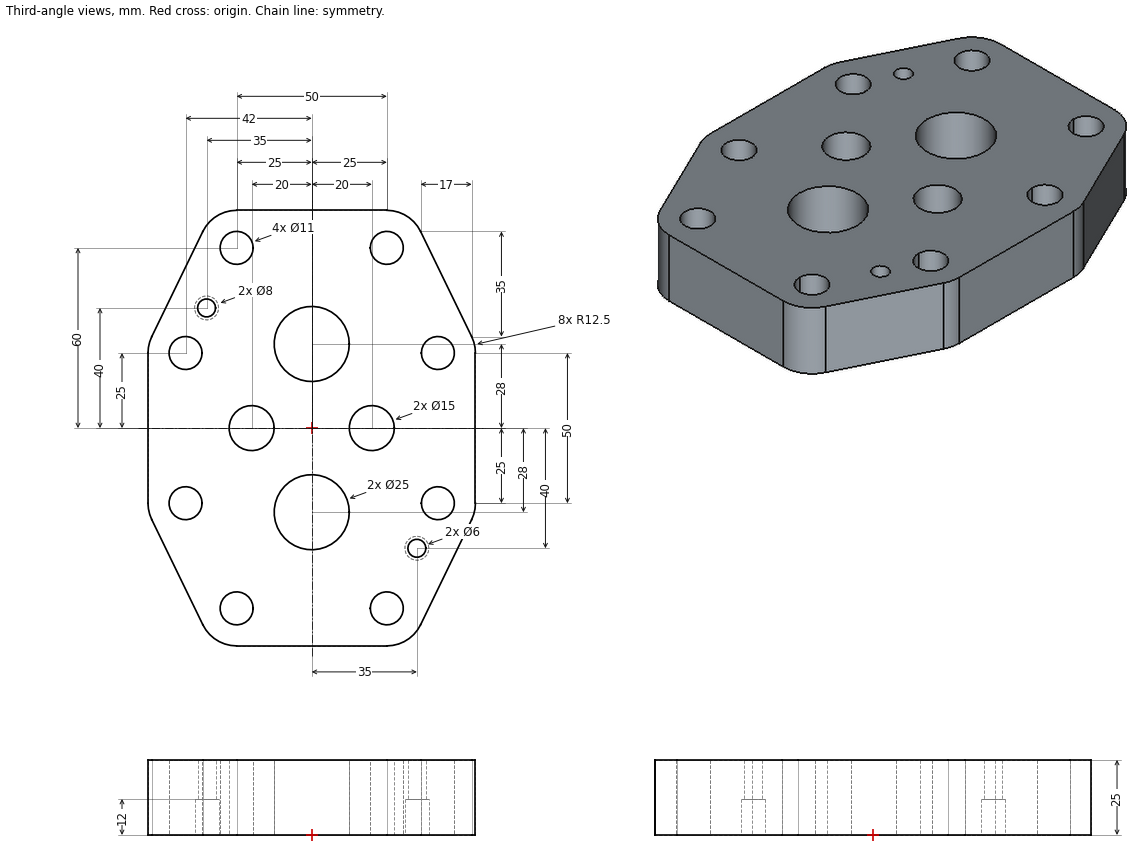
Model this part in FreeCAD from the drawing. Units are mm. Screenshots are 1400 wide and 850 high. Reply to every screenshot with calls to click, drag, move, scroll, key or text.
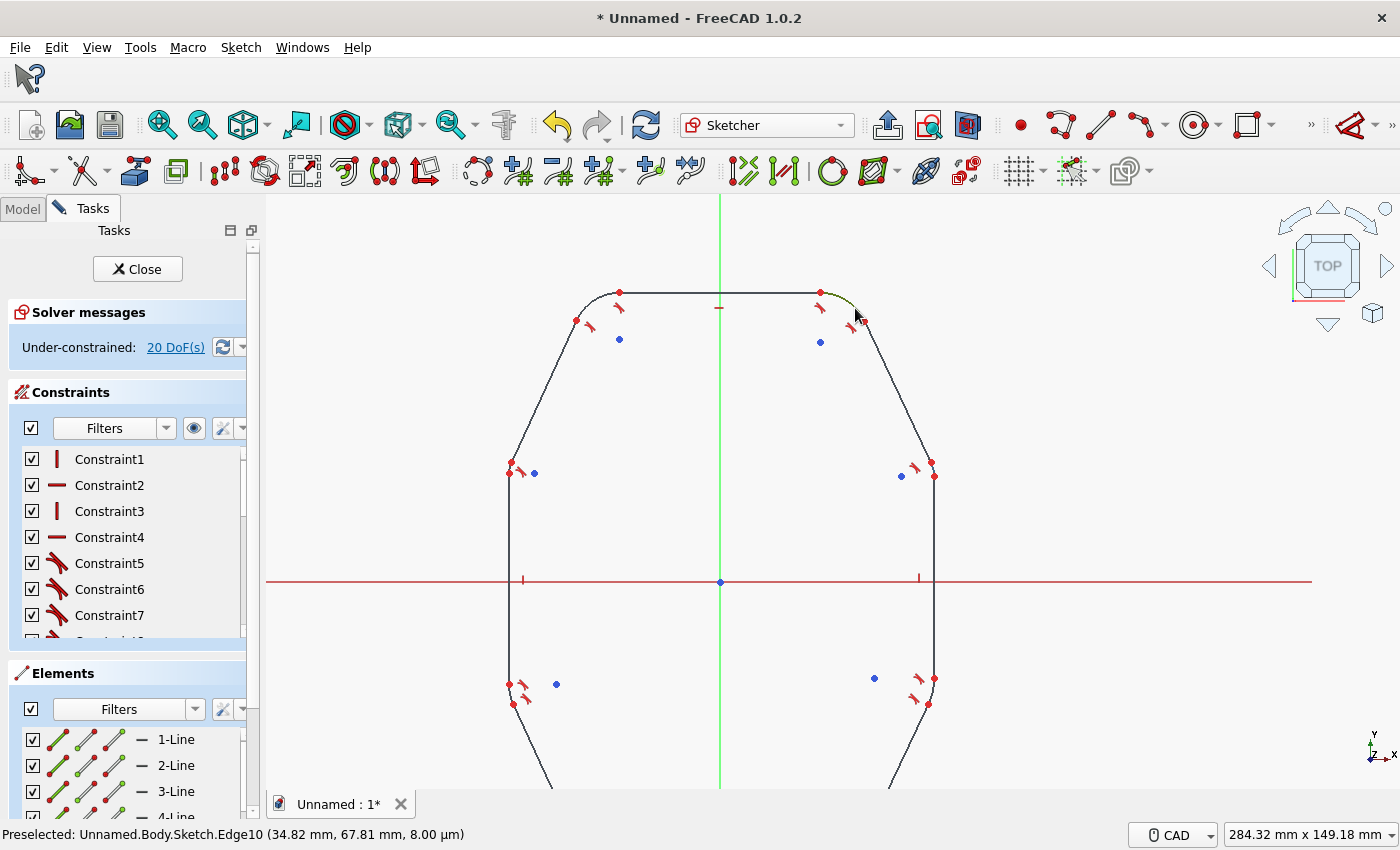
click(604, 296)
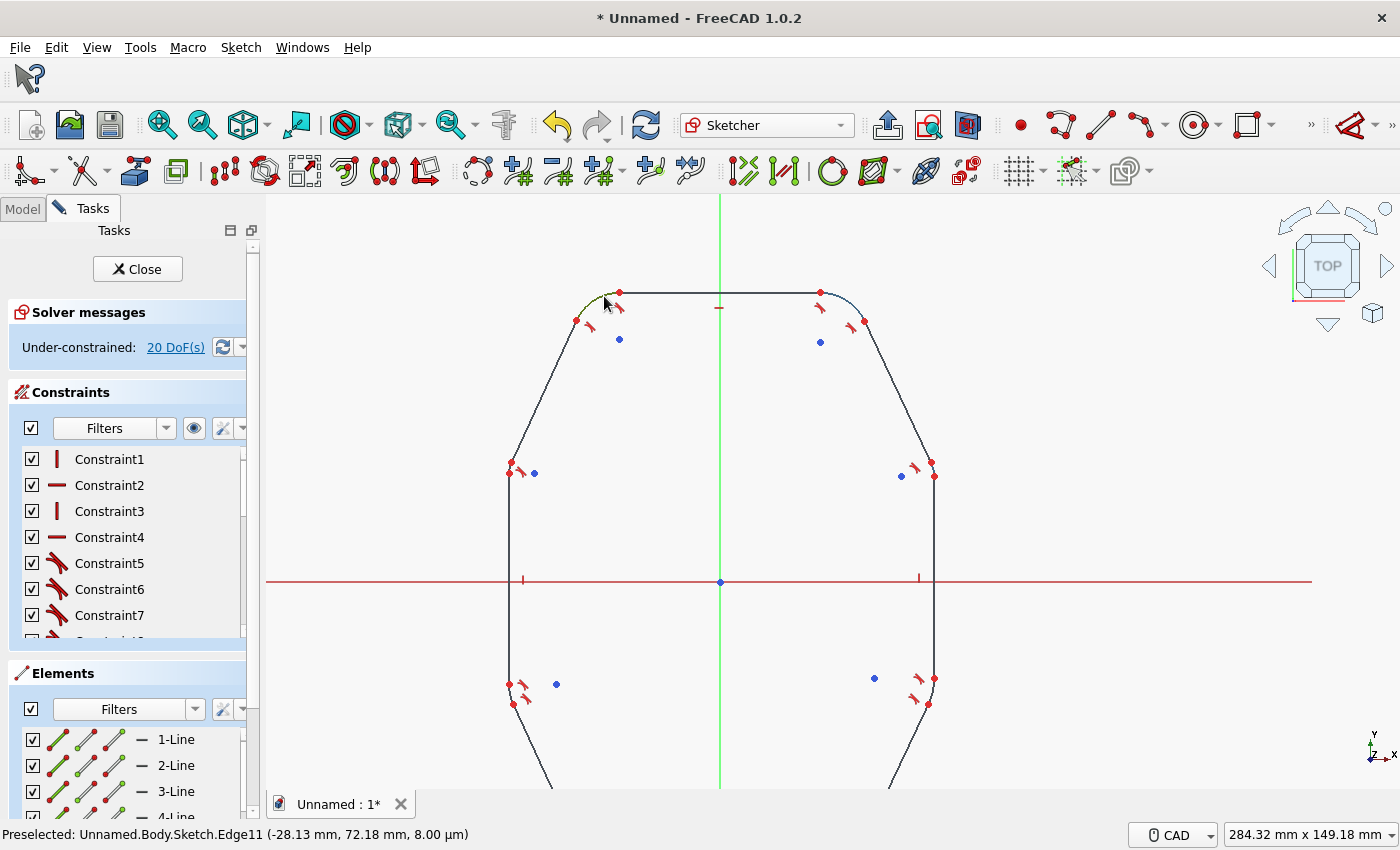
scroll(510, 468, up, 5)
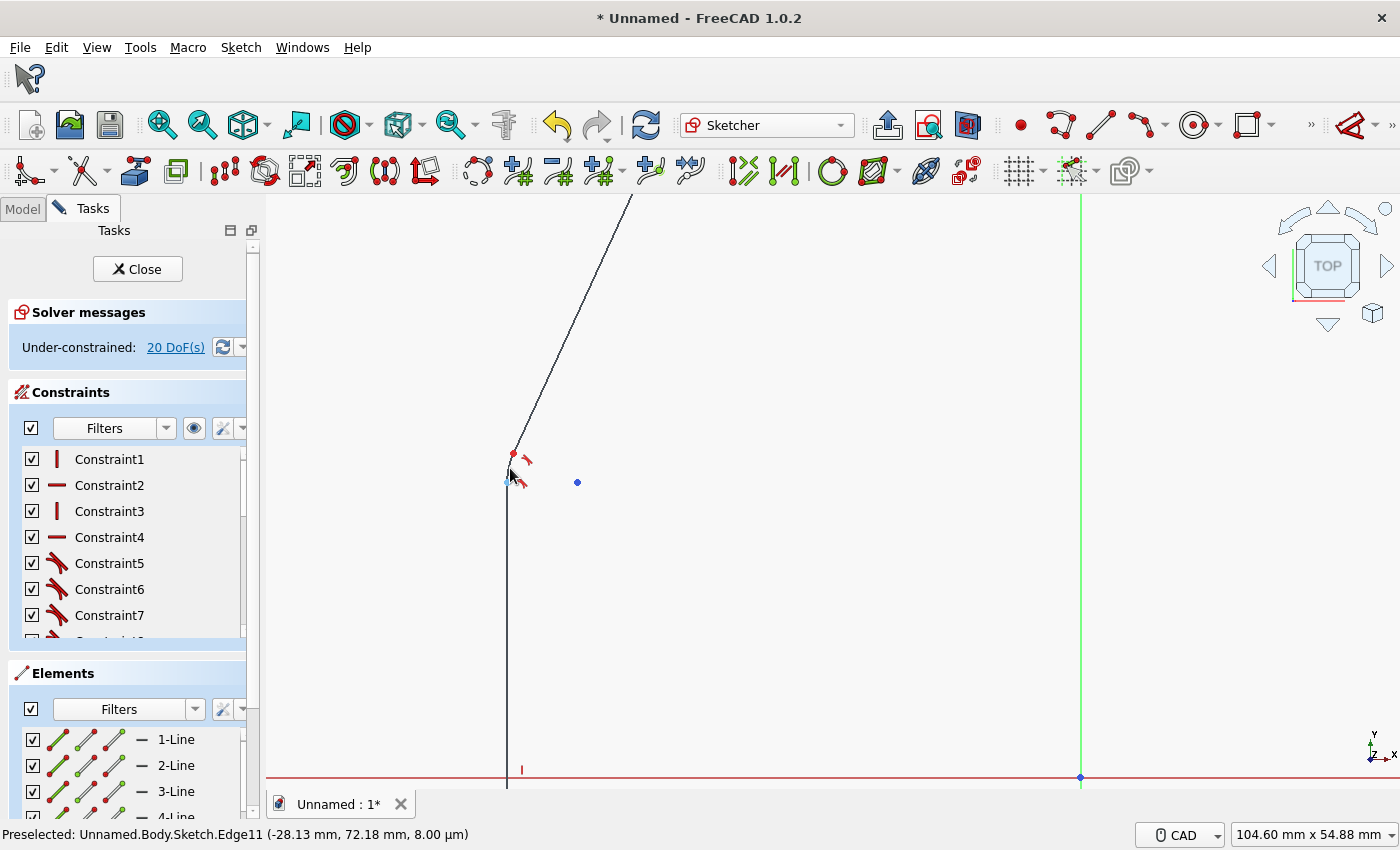
click(509, 468)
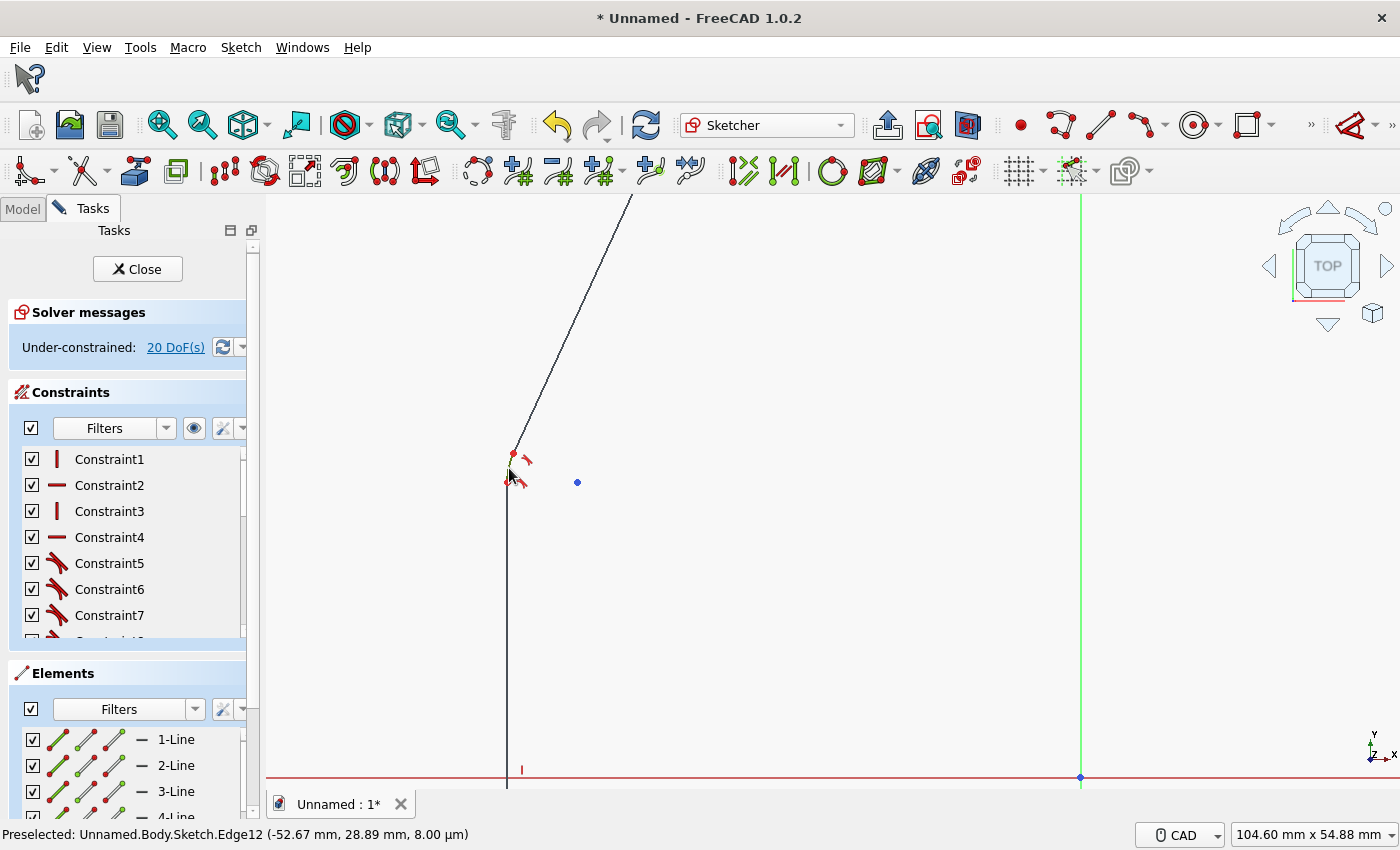
scroll(661, 398, down, 7)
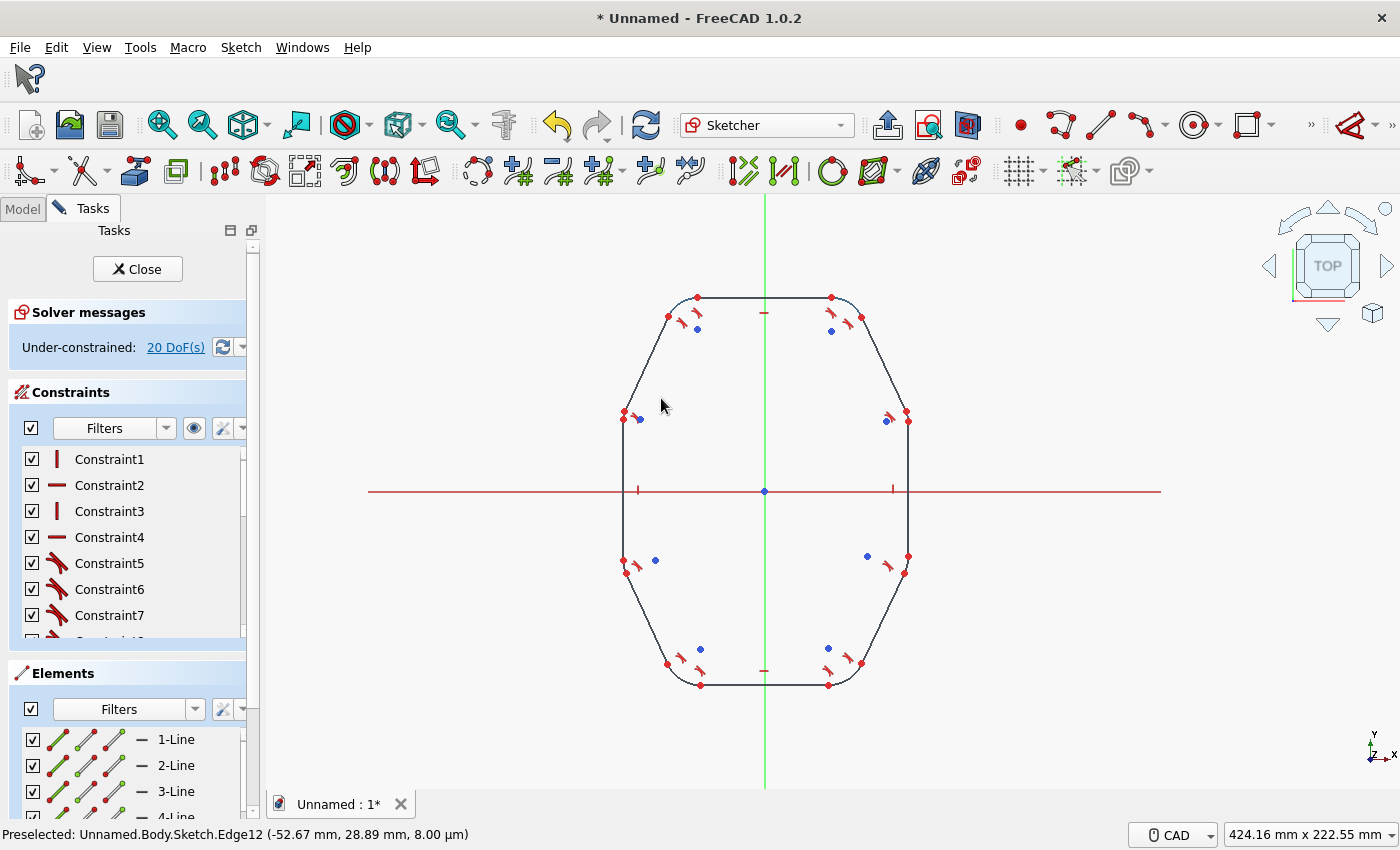
scroll(624, 565, up, 7)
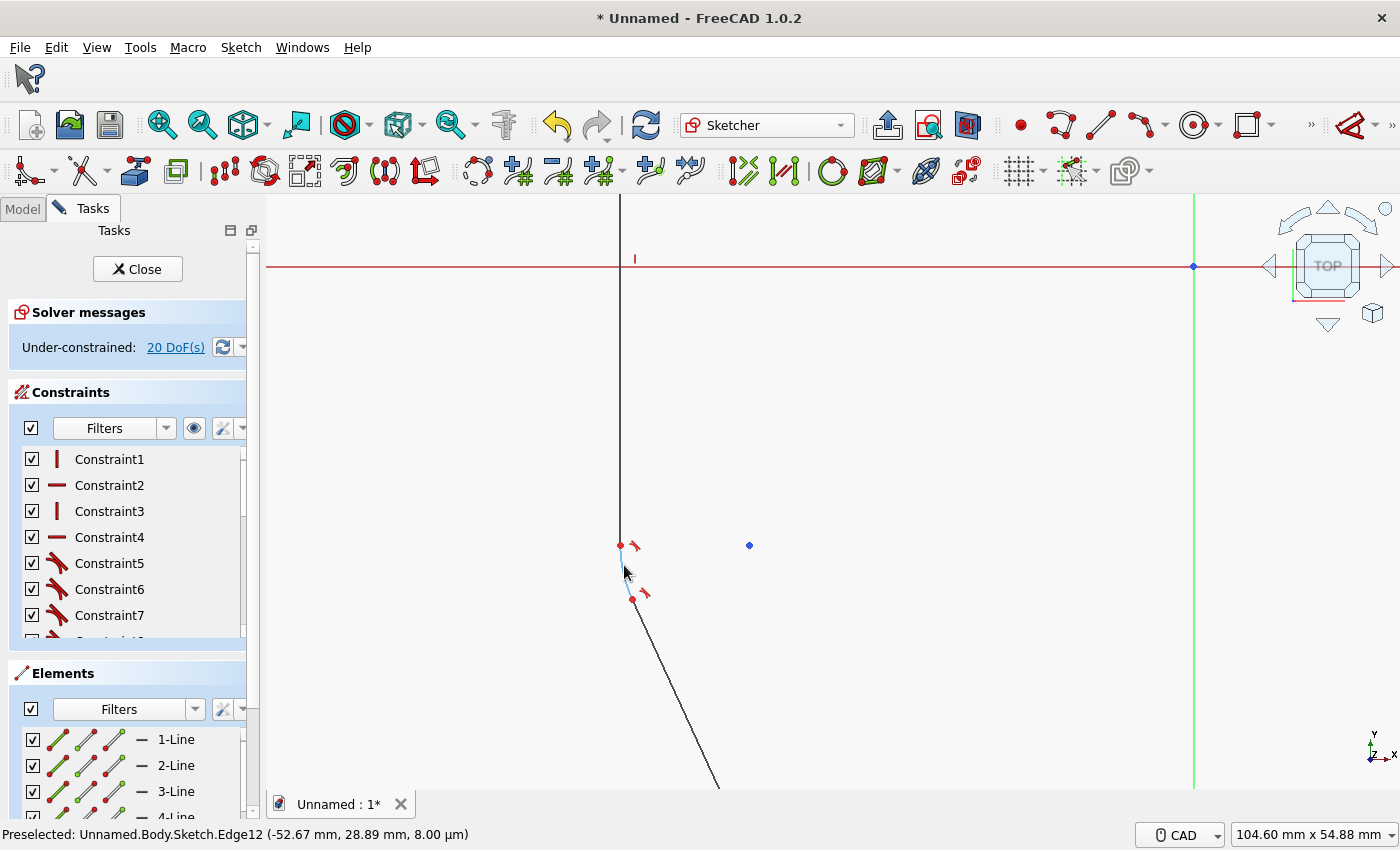
click(621, 562)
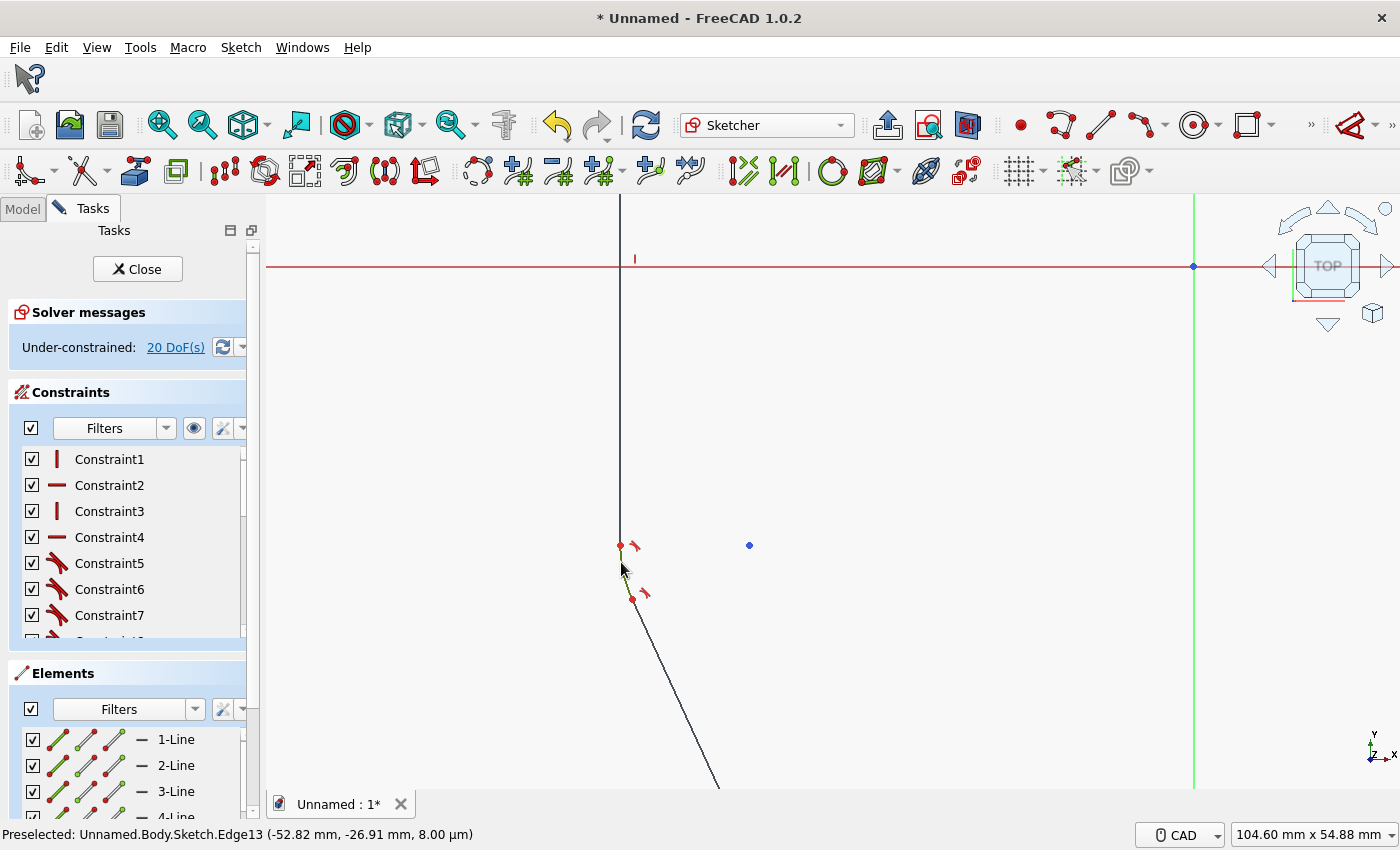
scroll(624, 565, down, 7)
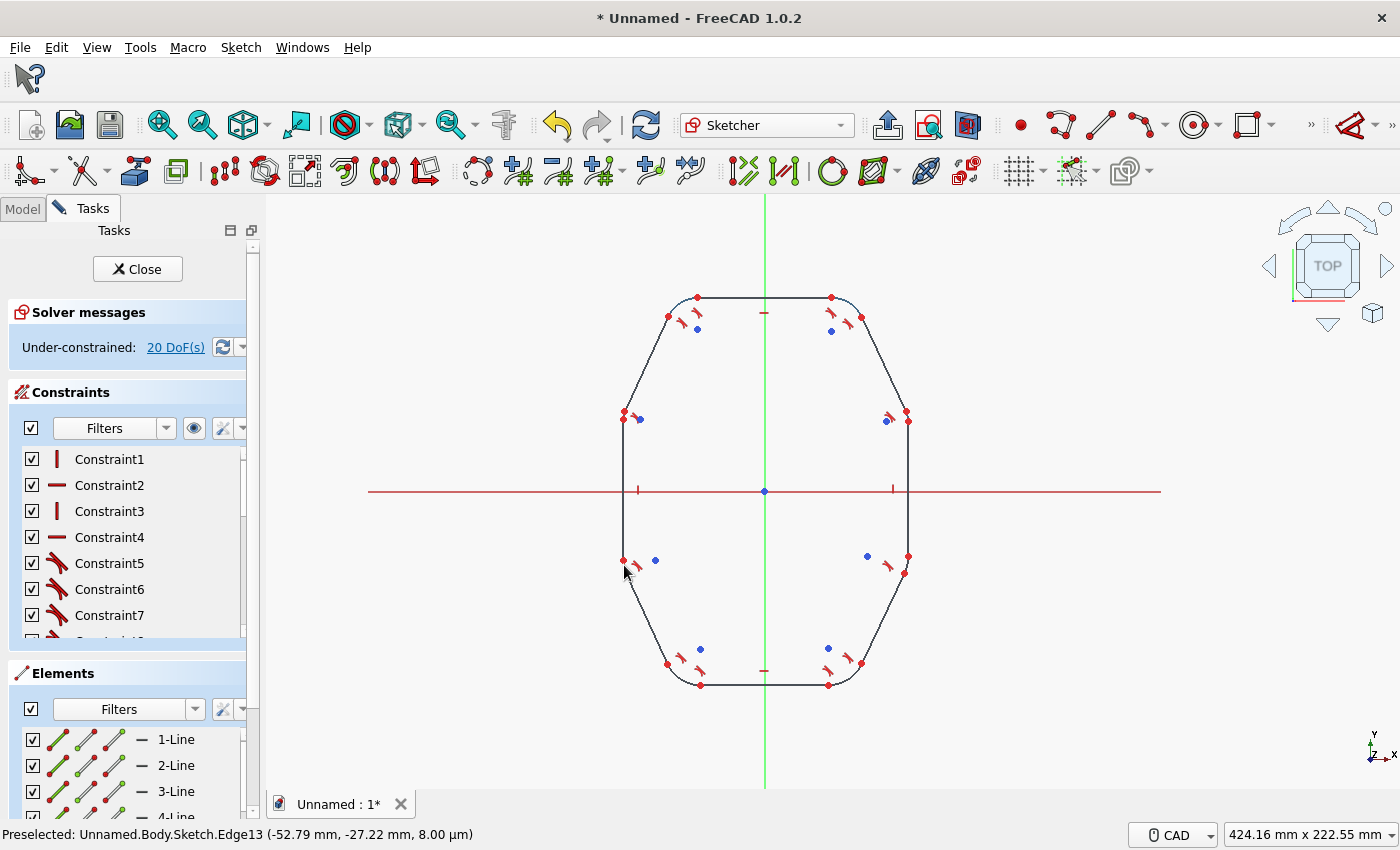
click(675, 674)